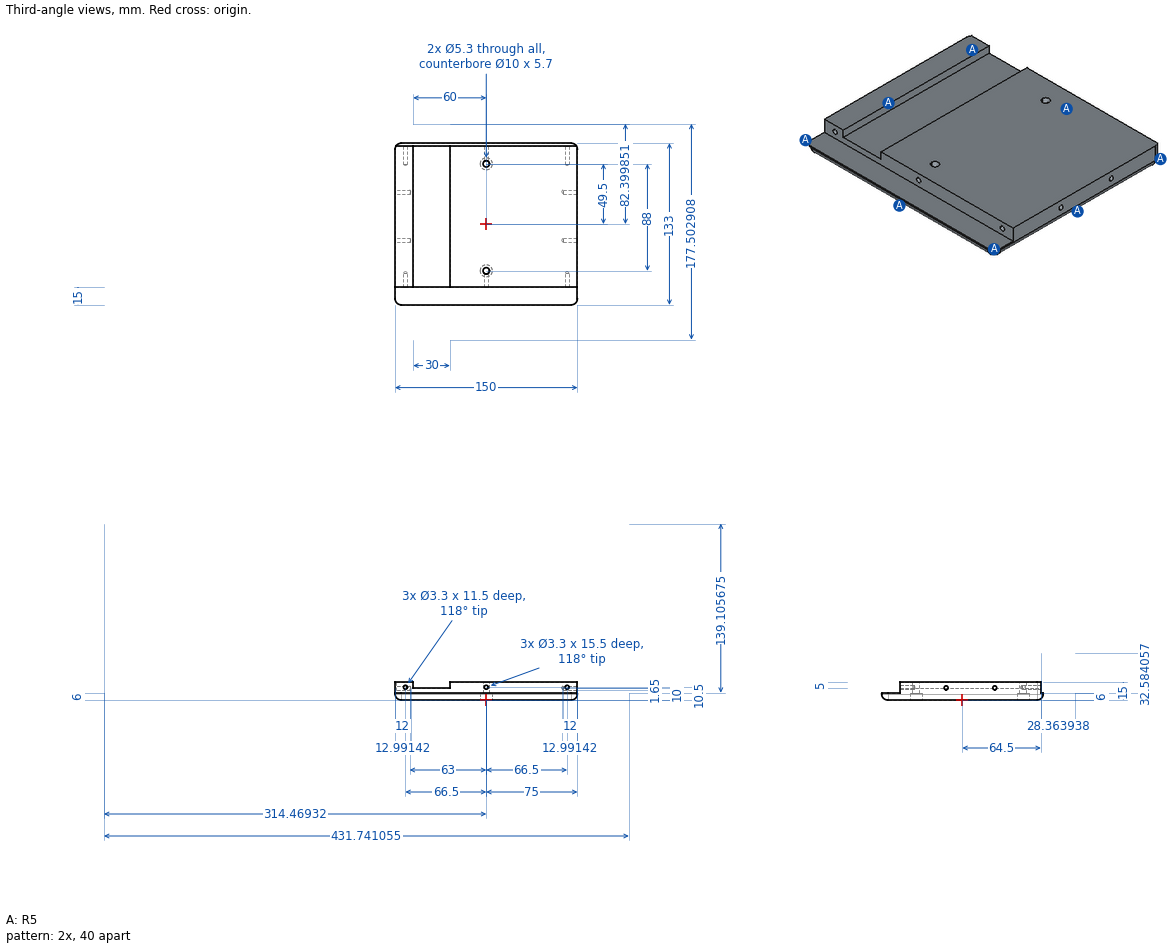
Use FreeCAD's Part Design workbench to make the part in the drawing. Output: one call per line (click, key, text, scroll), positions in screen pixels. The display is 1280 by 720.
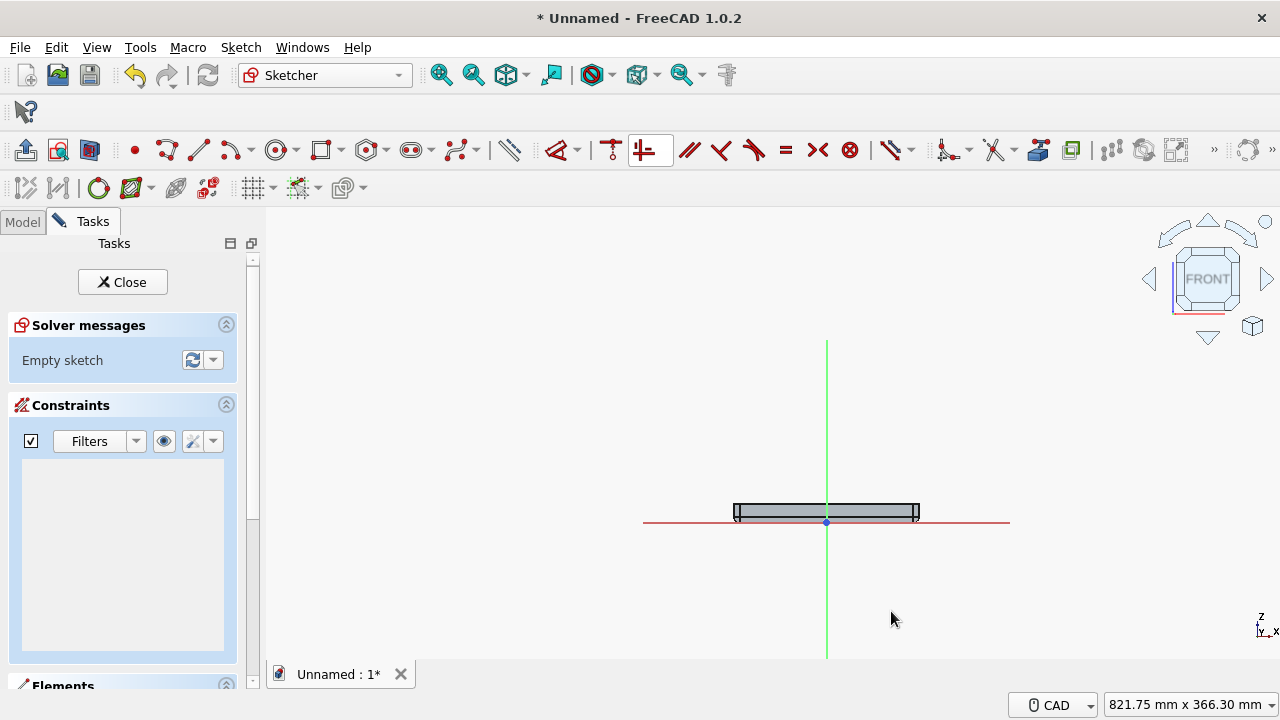
click(322, 150)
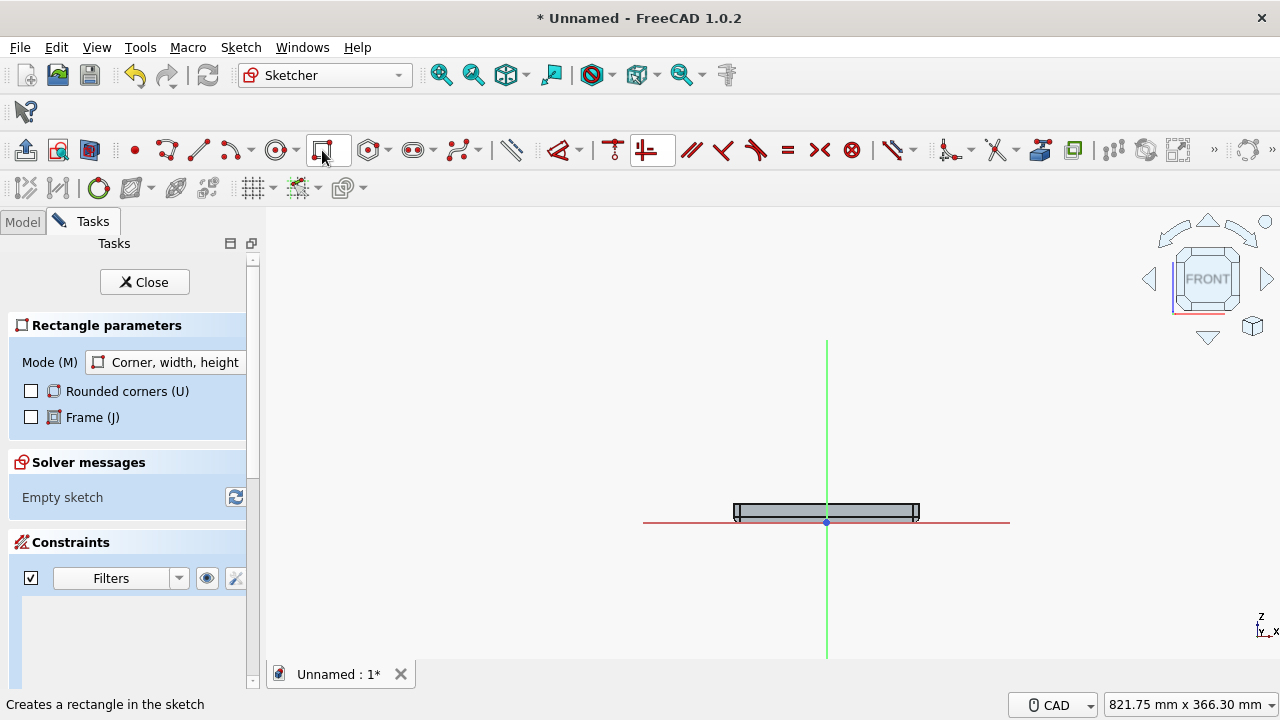
click(438, 344)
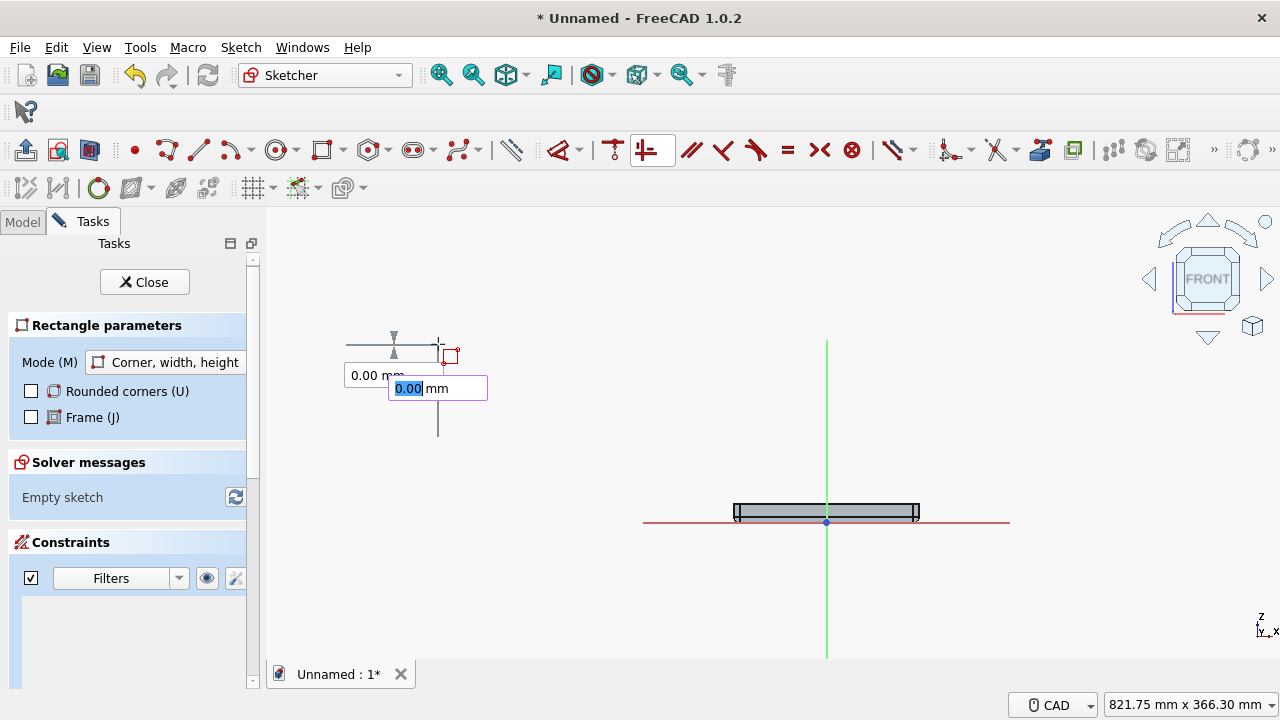
scroll(971, 516, up, 4)
move(971, 514)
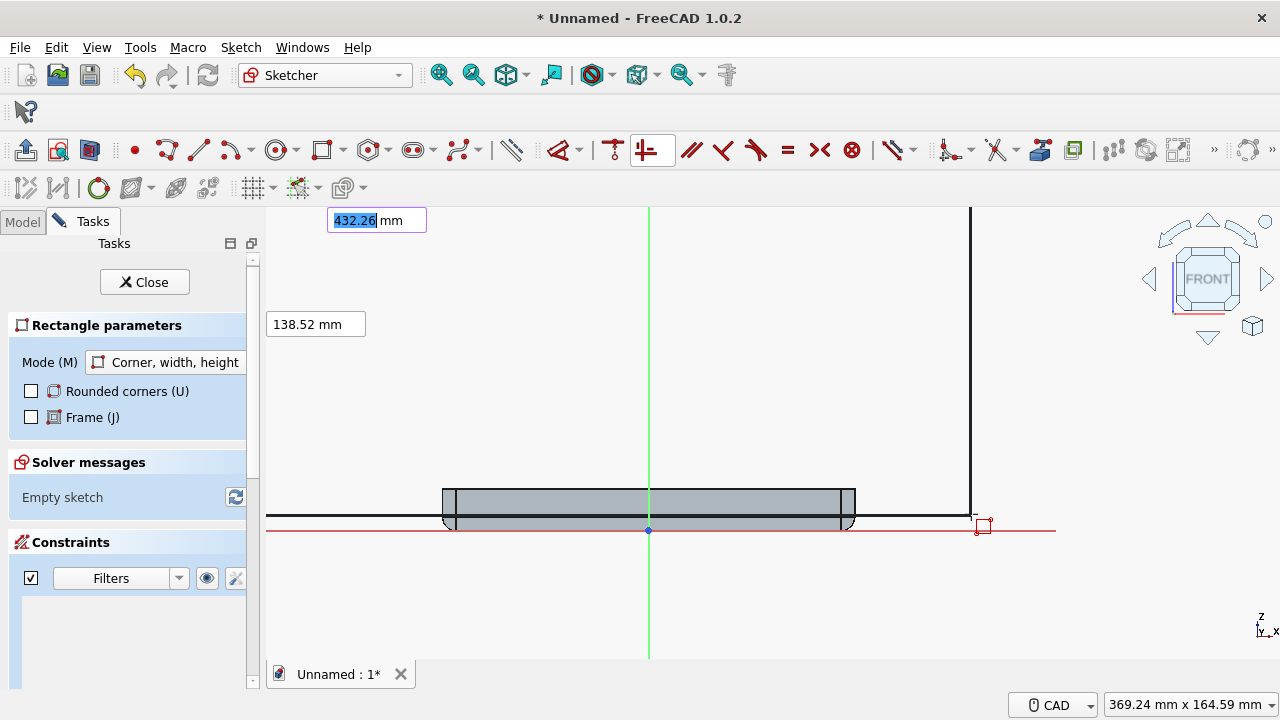
text(431.741055)
key(Tab)
text(139.105675)
key(Return)
key(Escape)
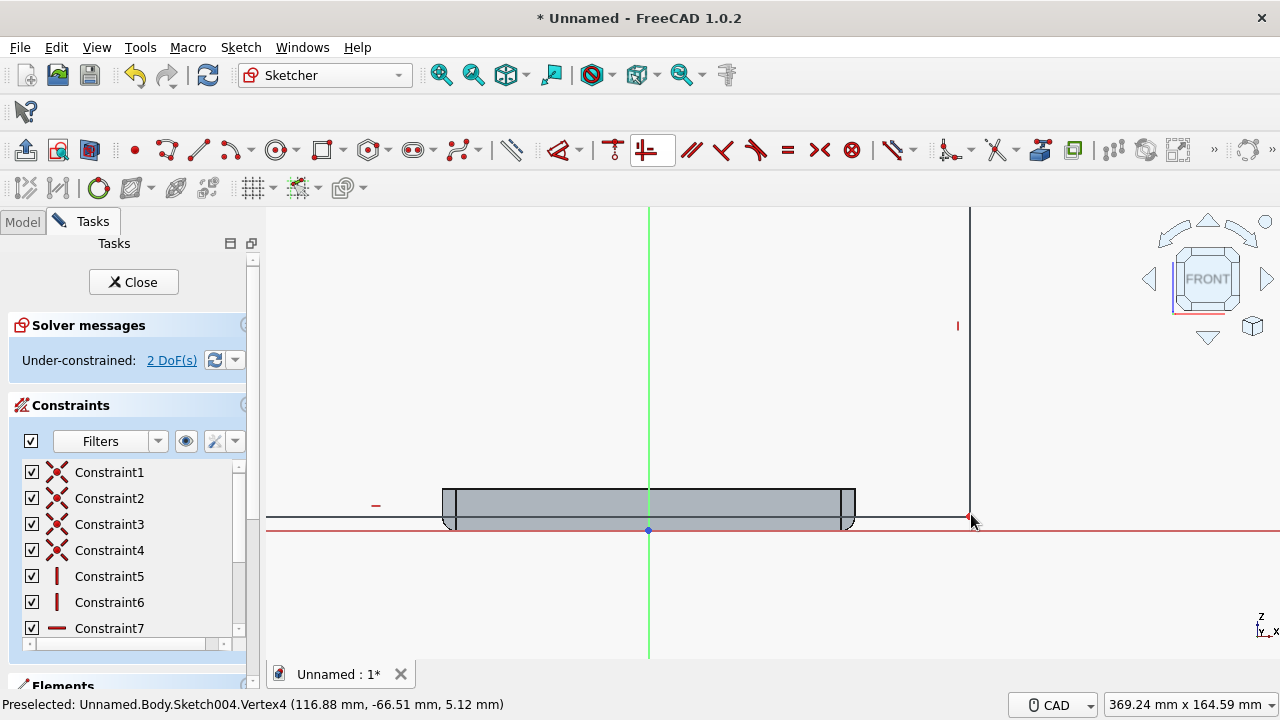
click(558, 150)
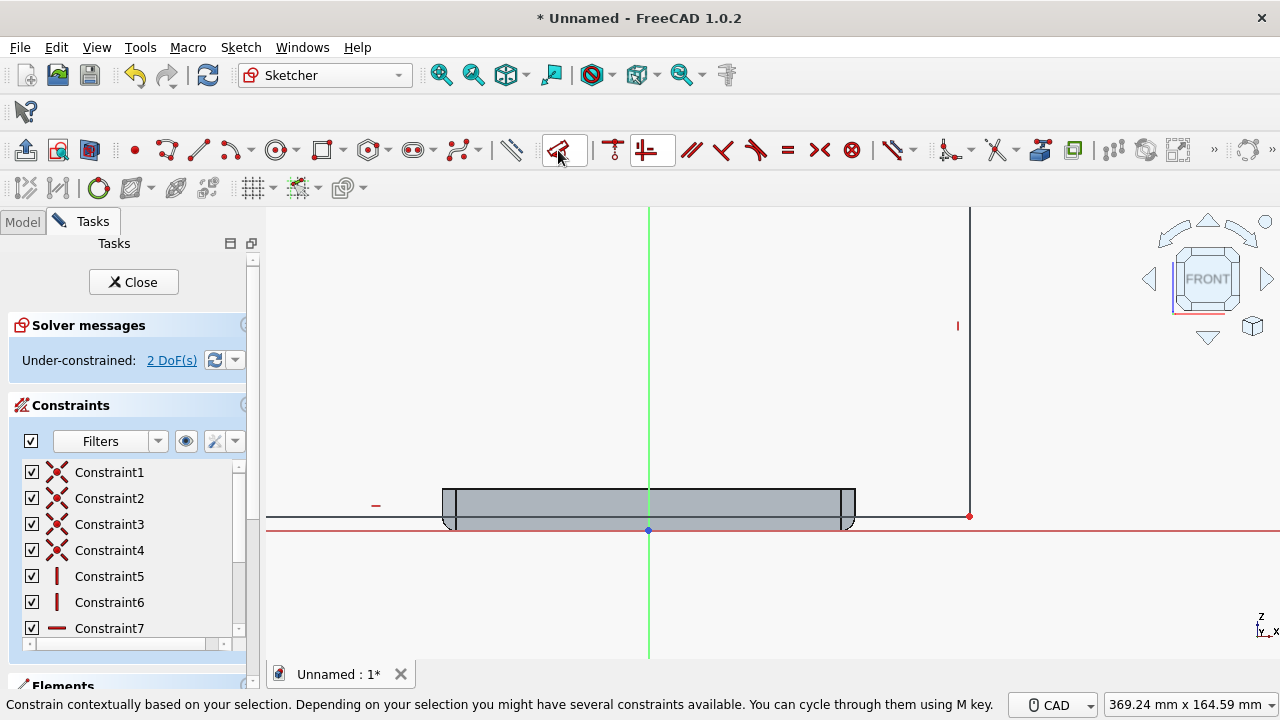
scroll(971, 516, down, 4)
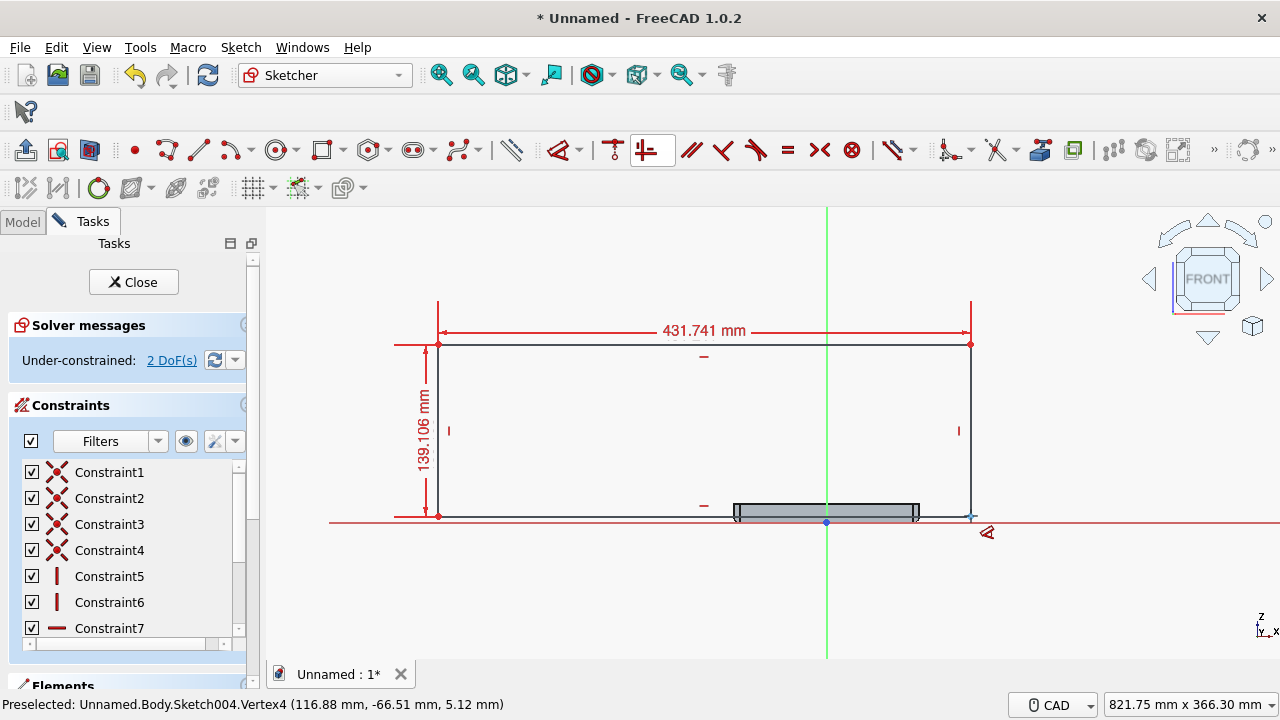
scroll(438, 517, up, 9)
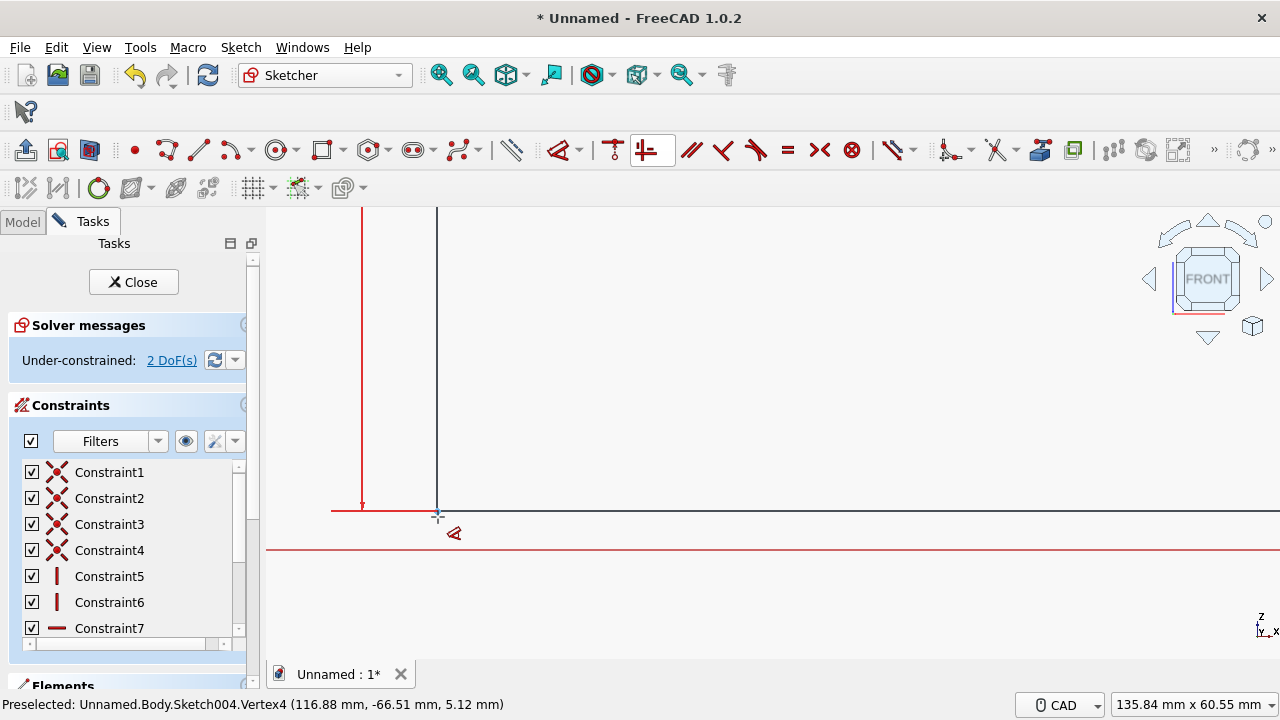
click(437, 511)
click(403, 531)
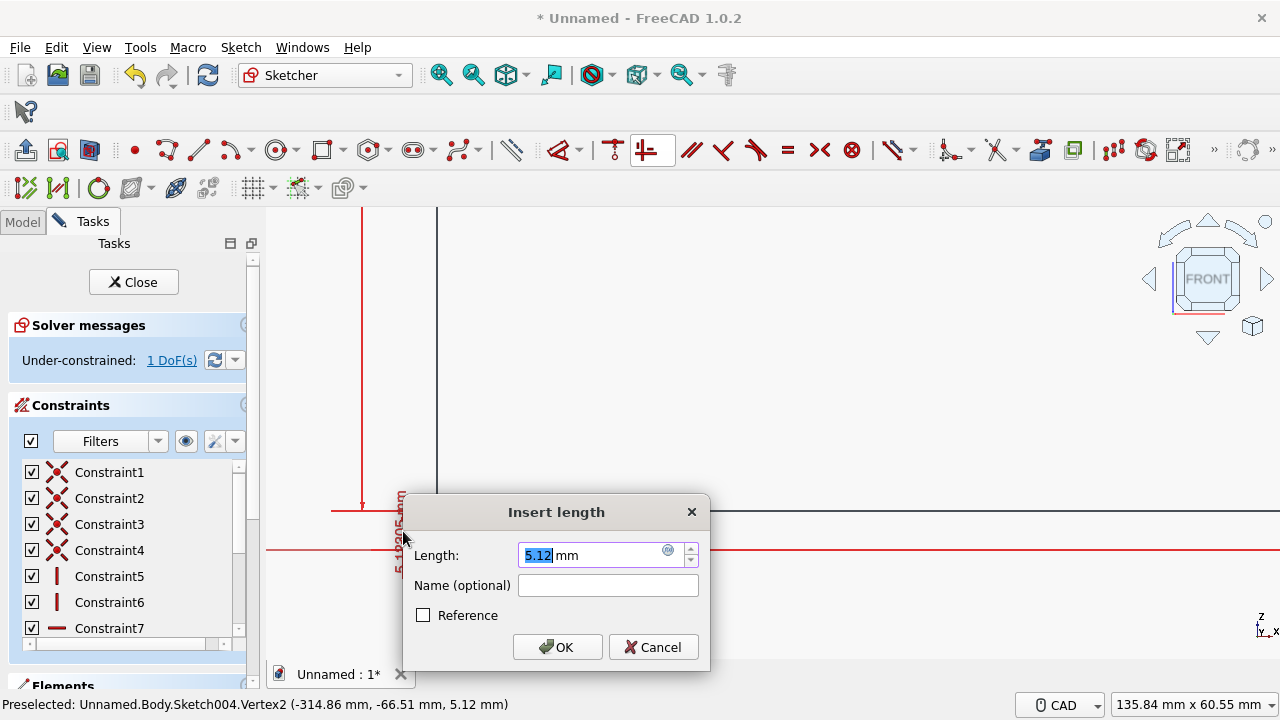
text(6)
key(Return)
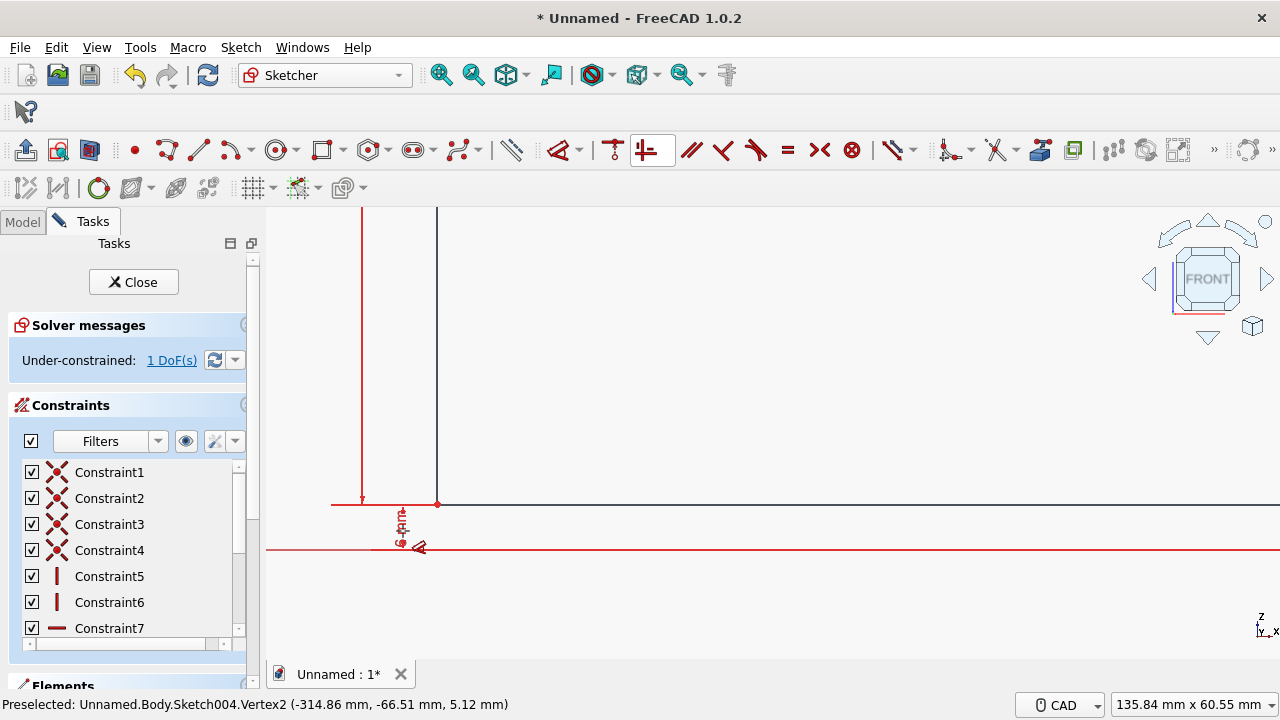
scroll(438, 517, down, 9)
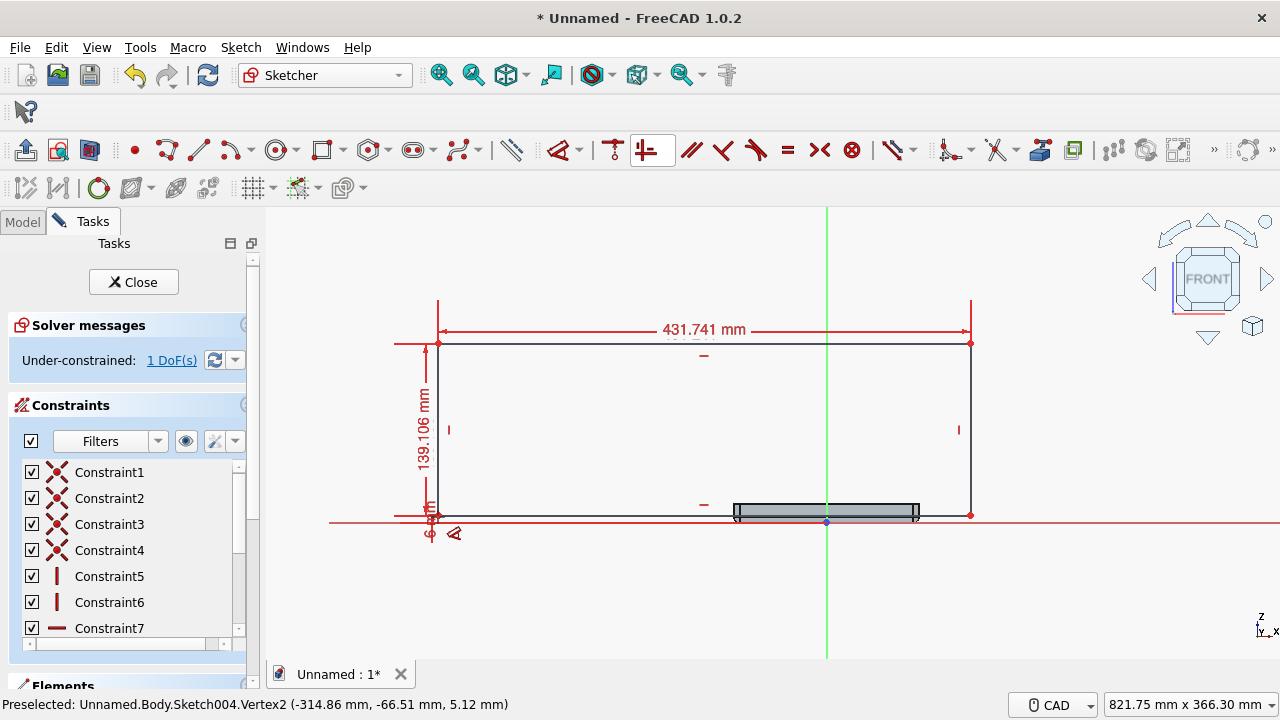
click(438, 344)
click(632, 557)